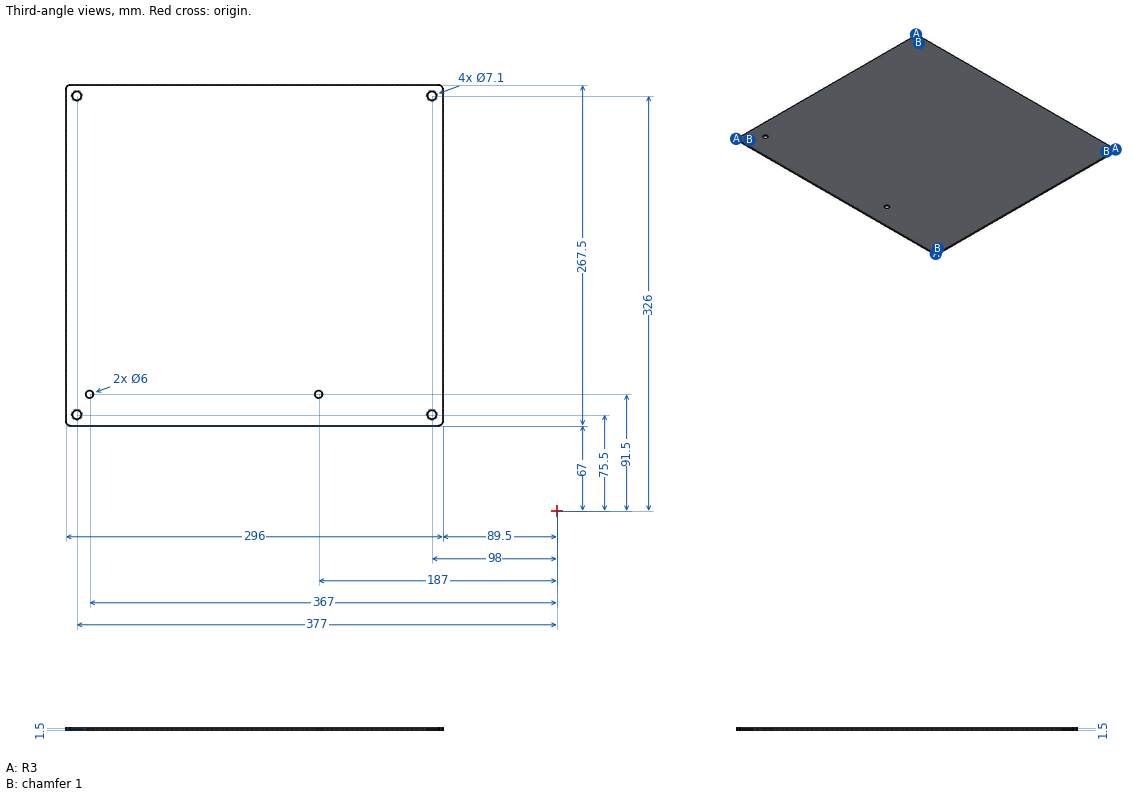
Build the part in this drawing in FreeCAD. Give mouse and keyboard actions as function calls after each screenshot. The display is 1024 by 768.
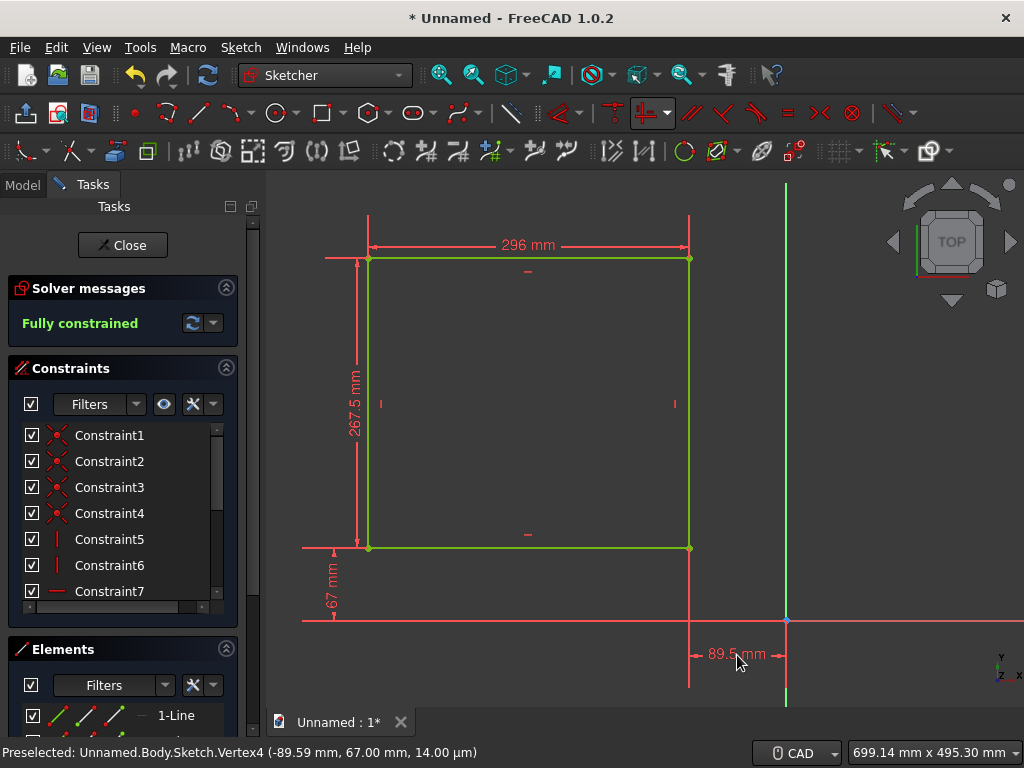
click(123, 245)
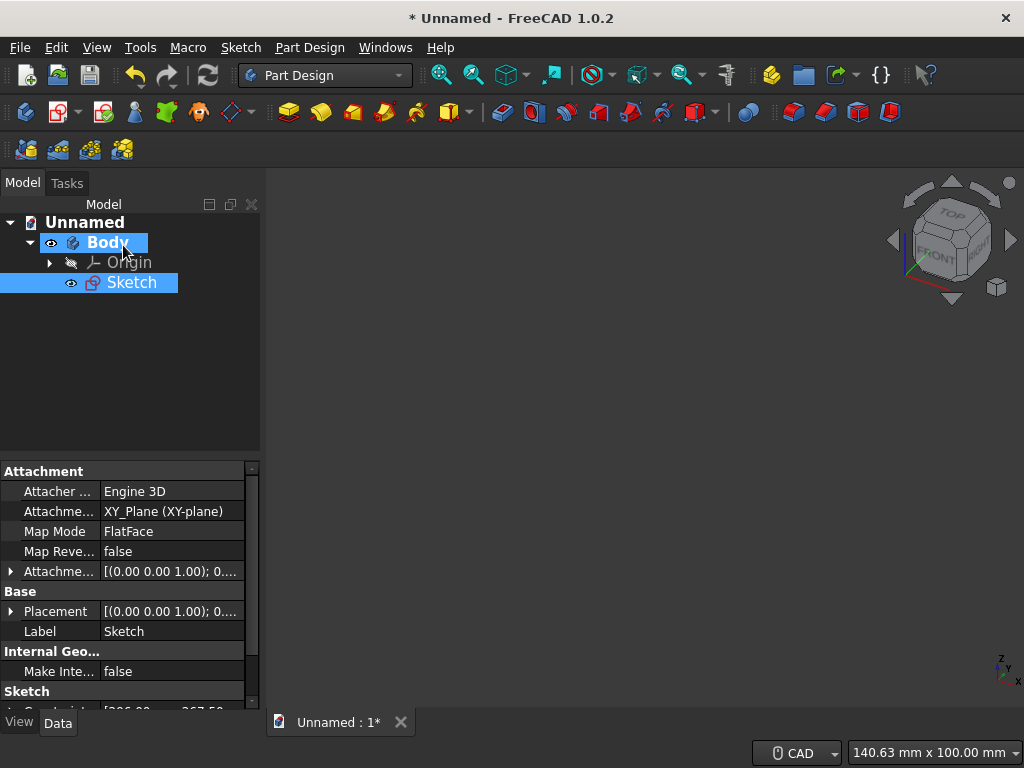
click(290, 112)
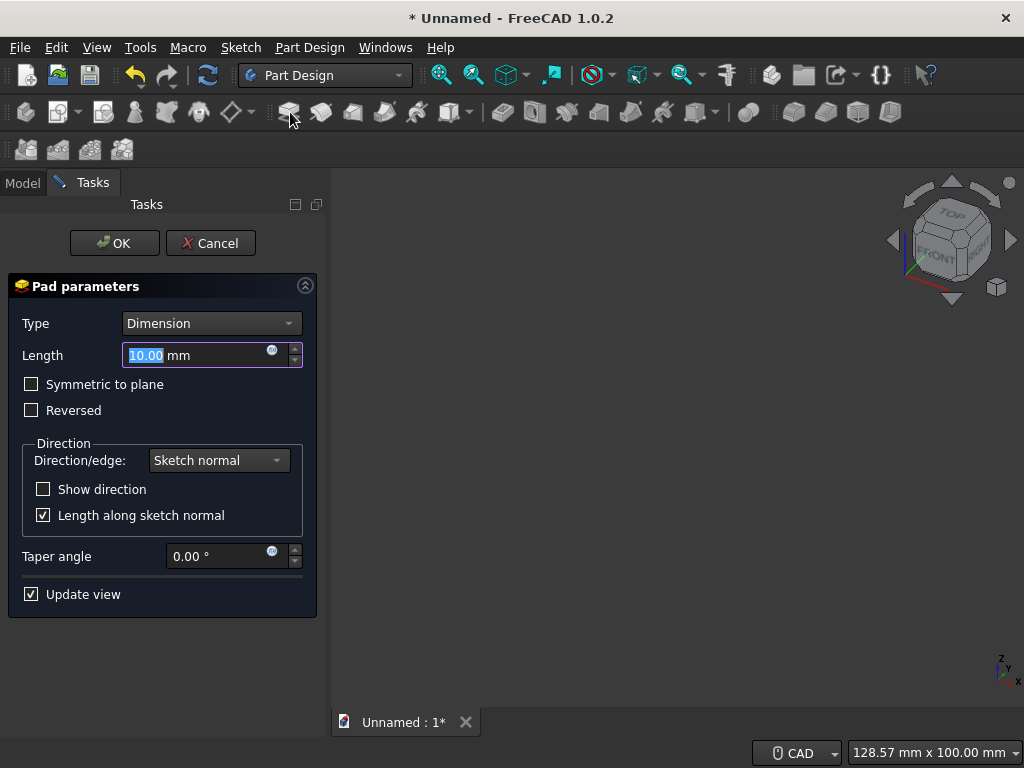
text(1.5)
key(Tab)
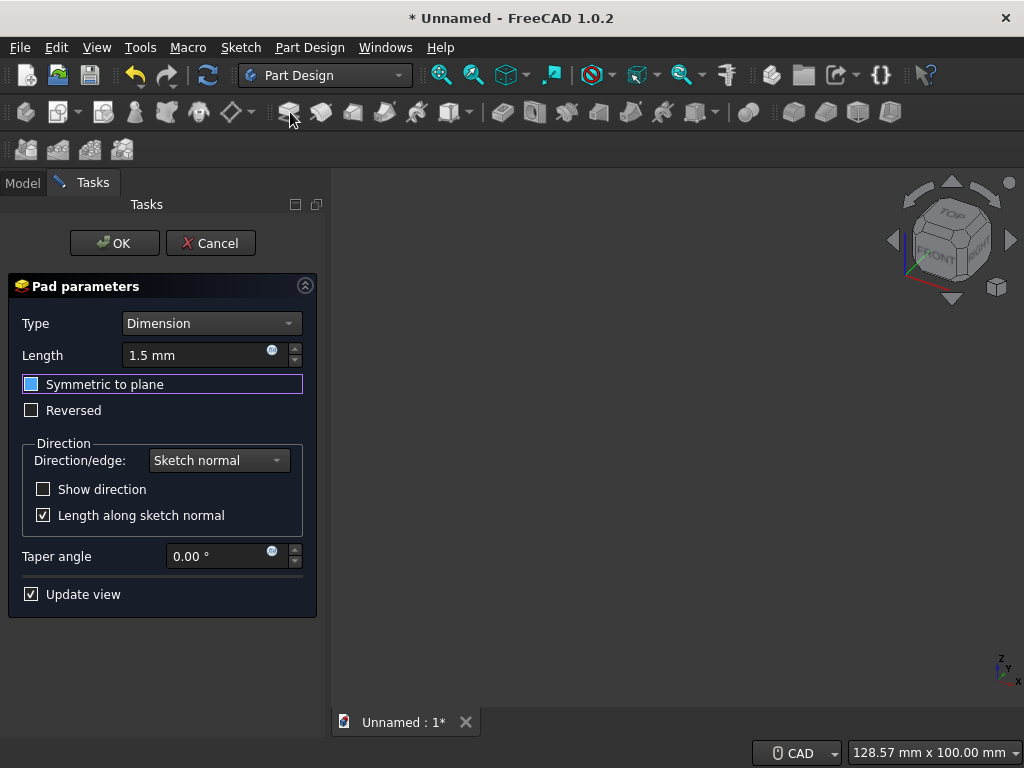
click(30, 410)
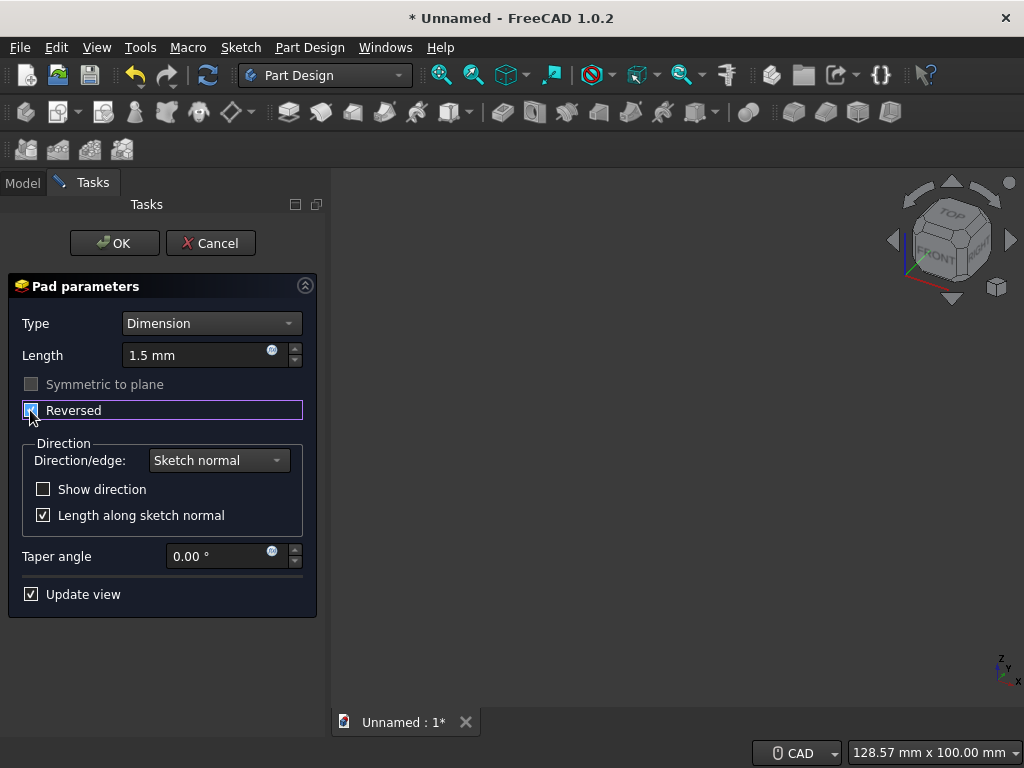
click(115, 243)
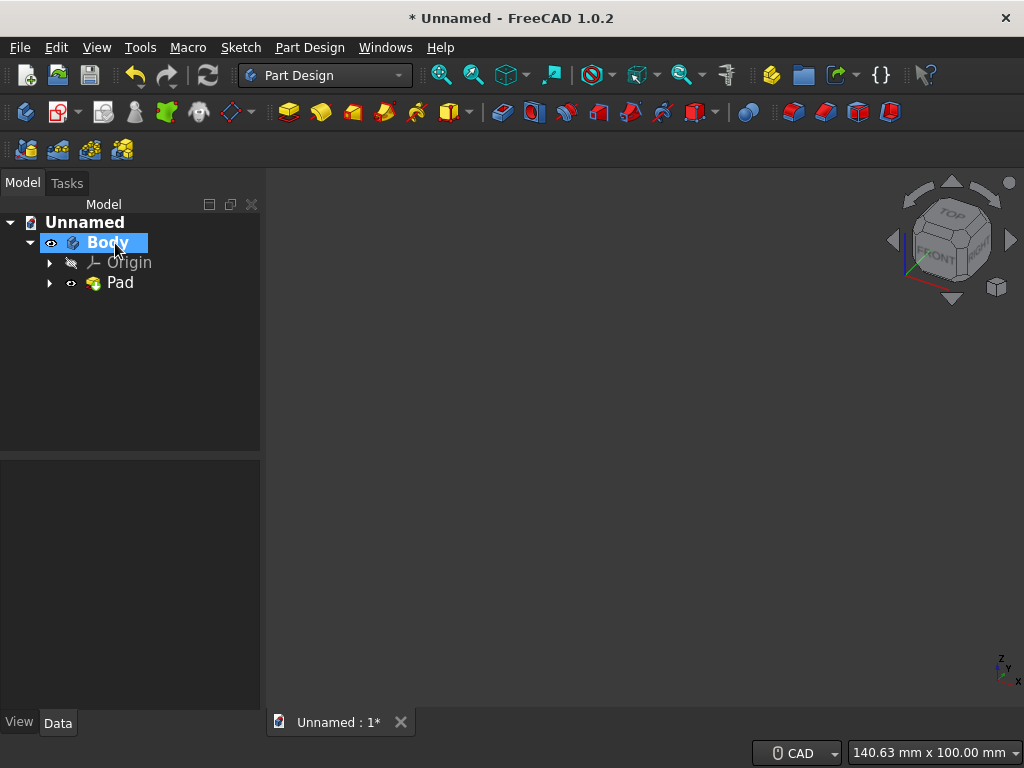
click(442, 76)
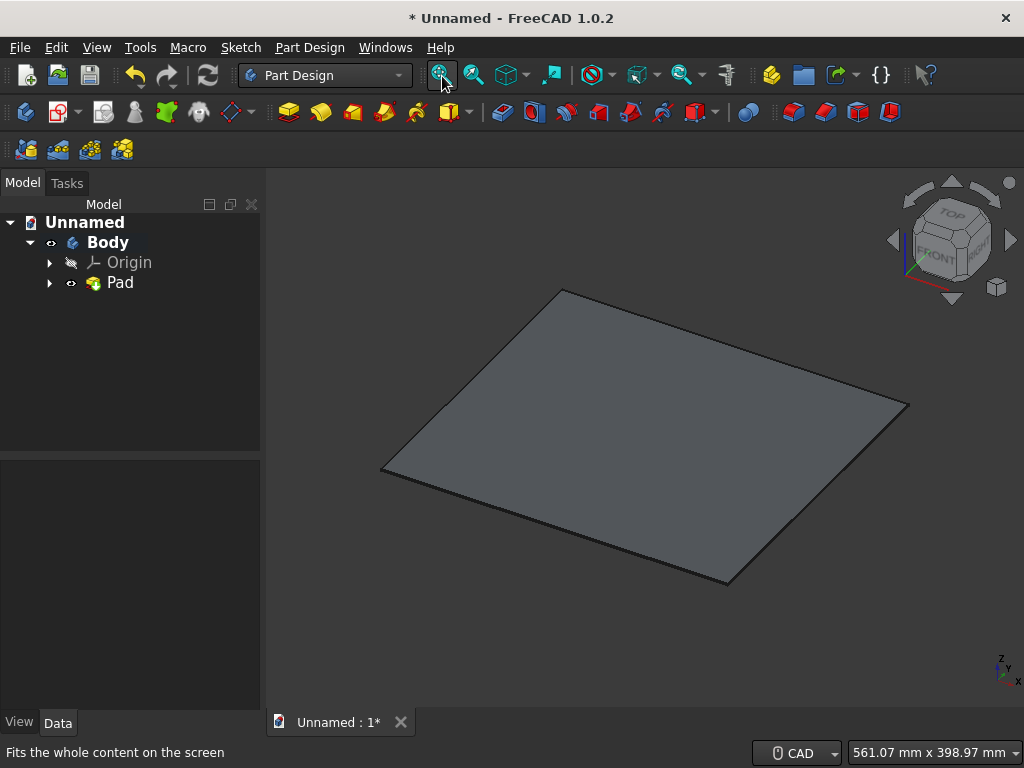
scroll(381, 469, up, 15)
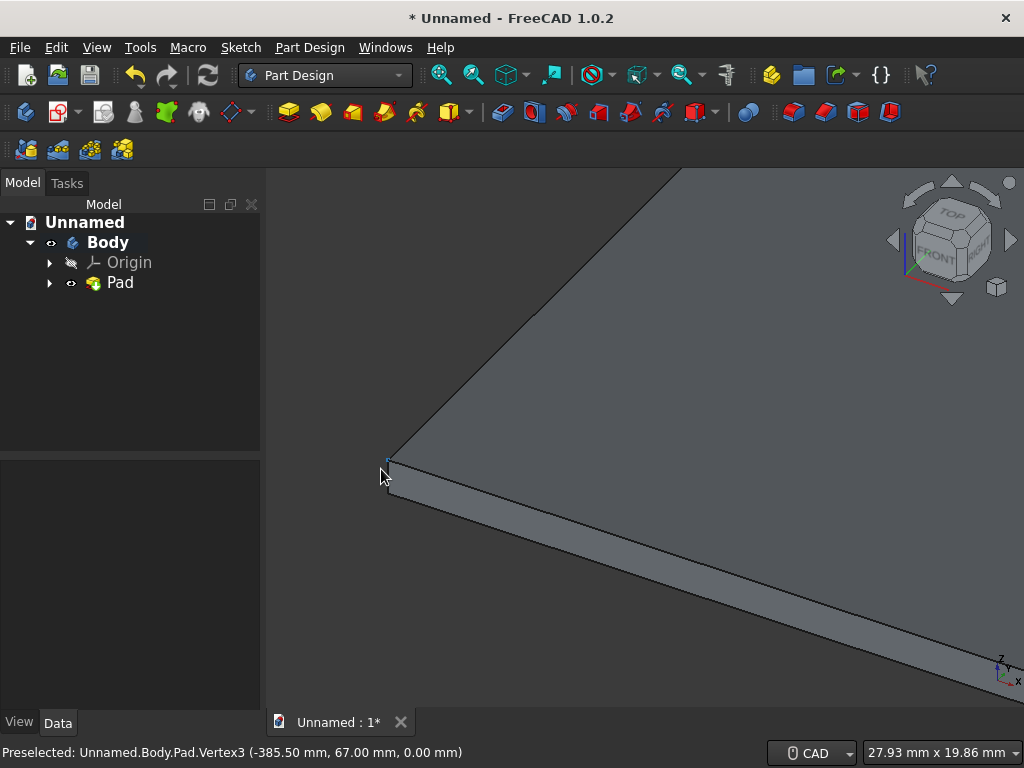
click(442, 76)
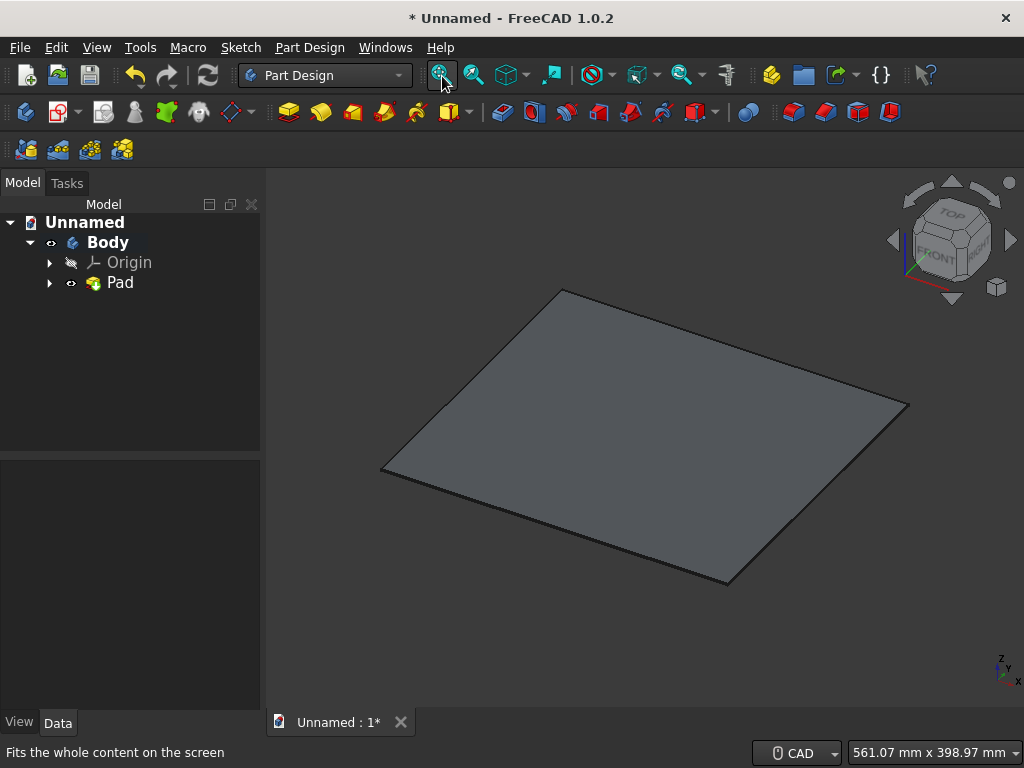
key(0)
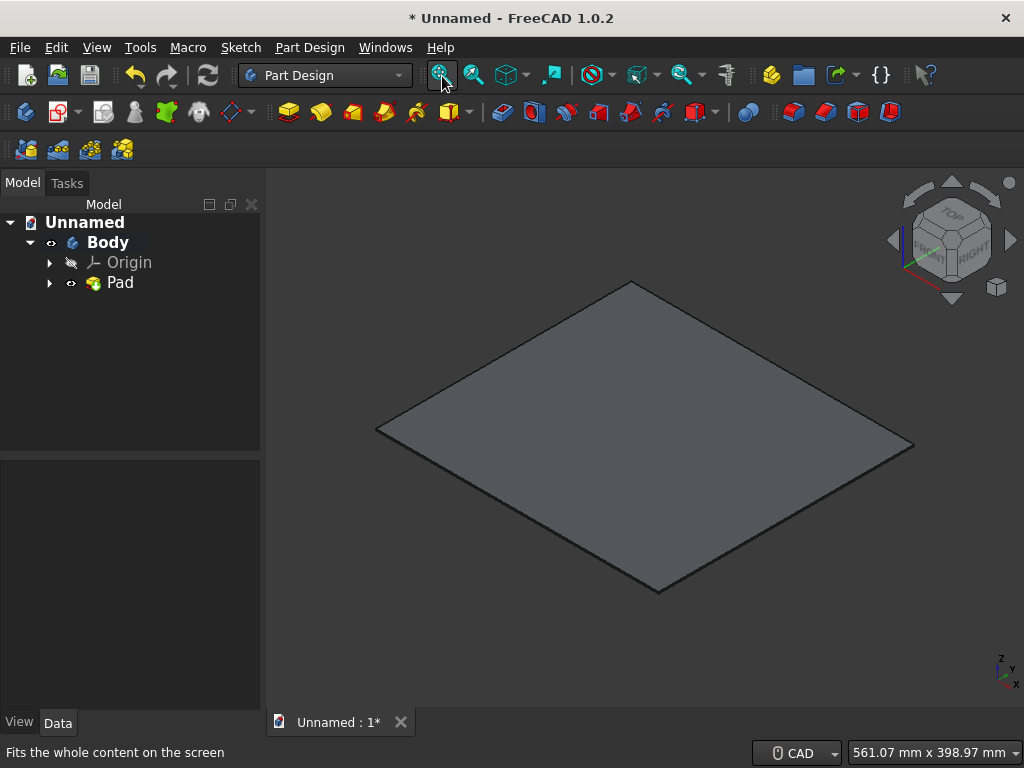
scroll(376, 429, up, 15)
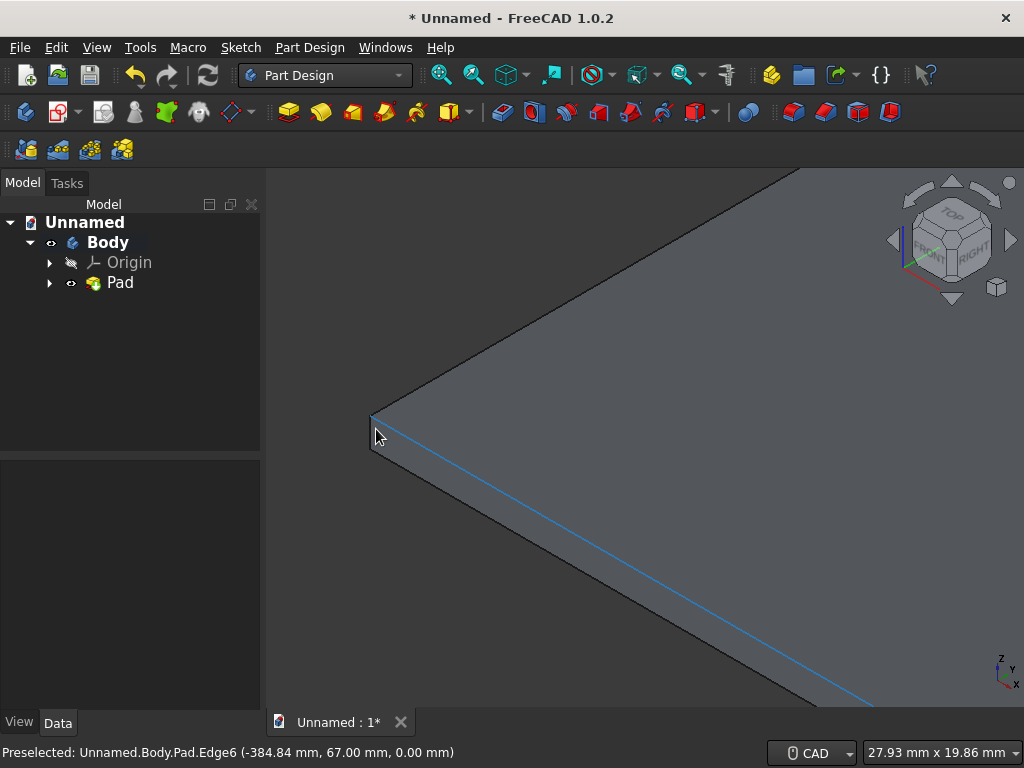
click(442, 76)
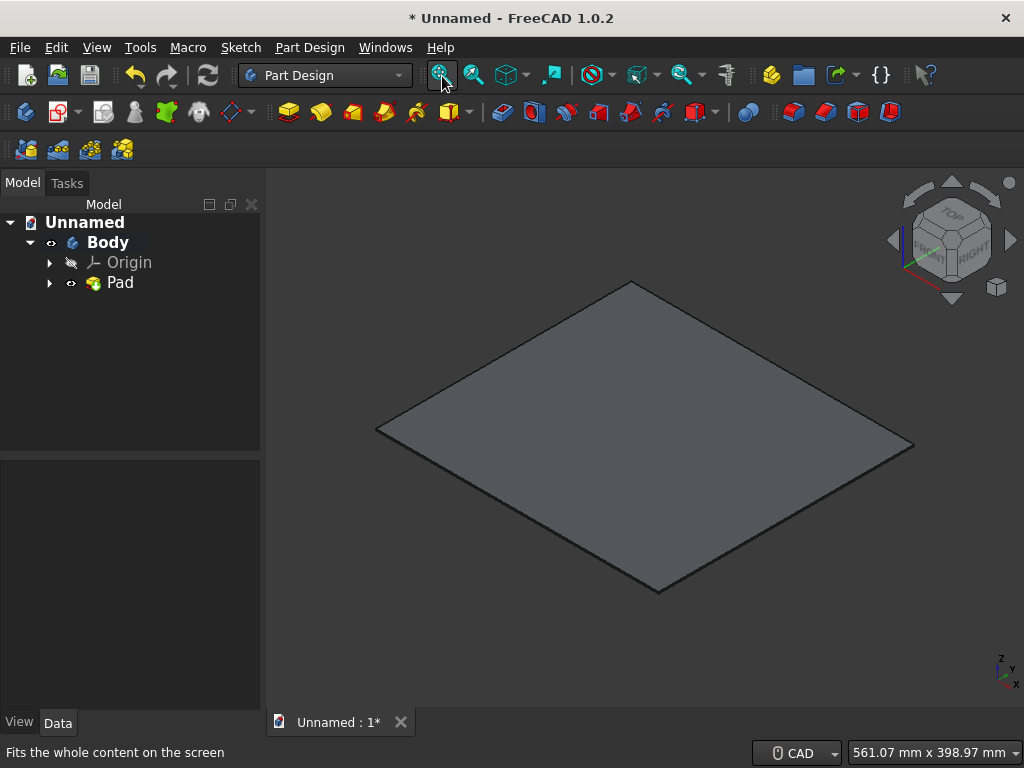
key(2)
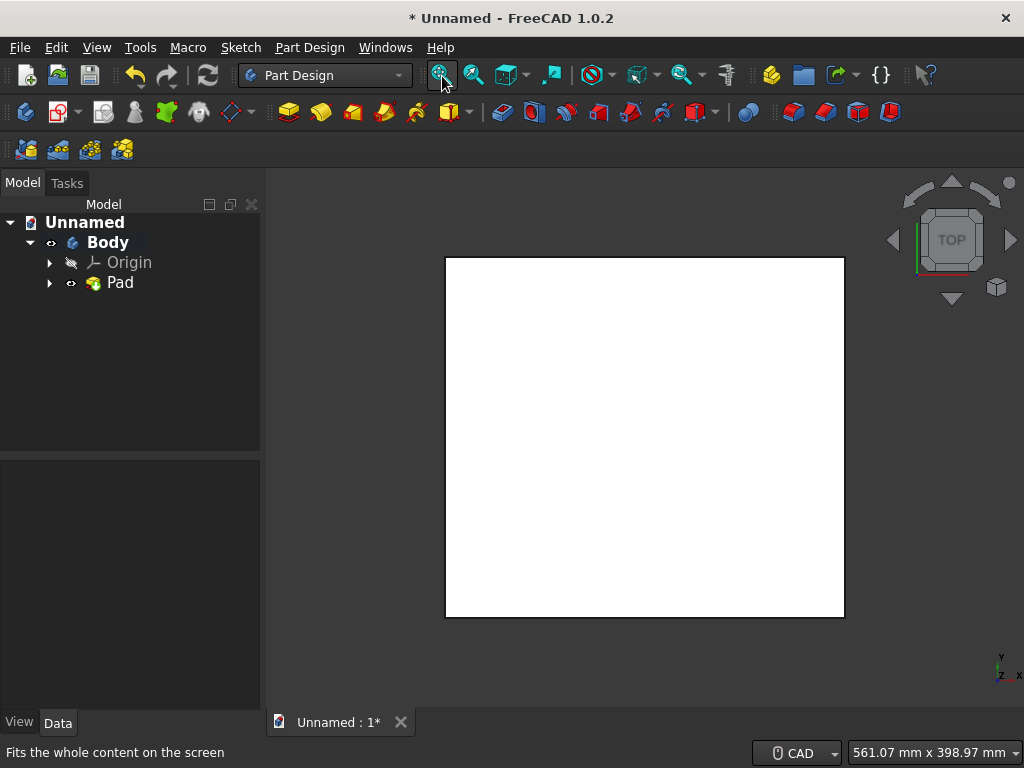
scroll(445, 617, up, 15)